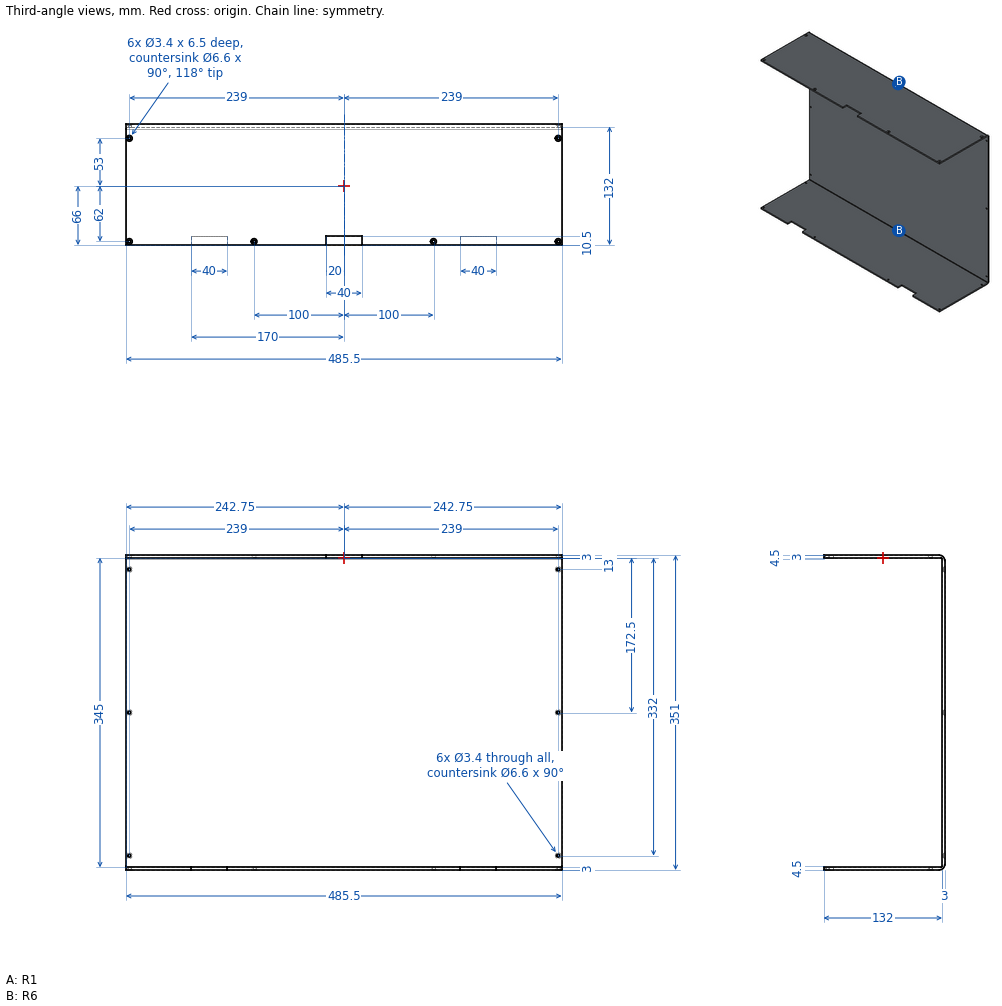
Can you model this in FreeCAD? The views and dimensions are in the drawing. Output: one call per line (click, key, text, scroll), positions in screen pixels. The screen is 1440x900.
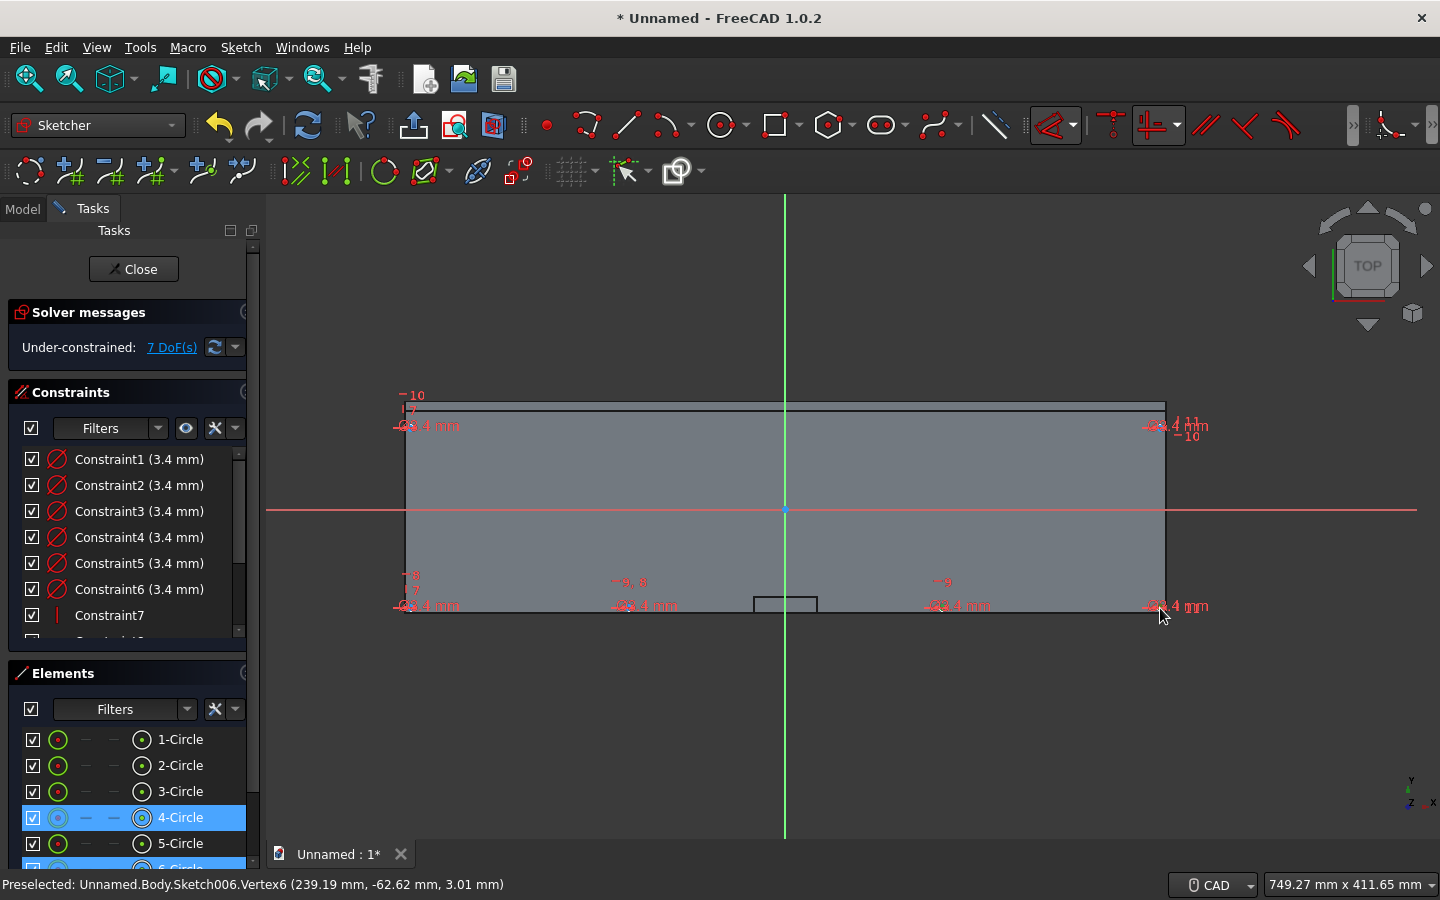
key(h)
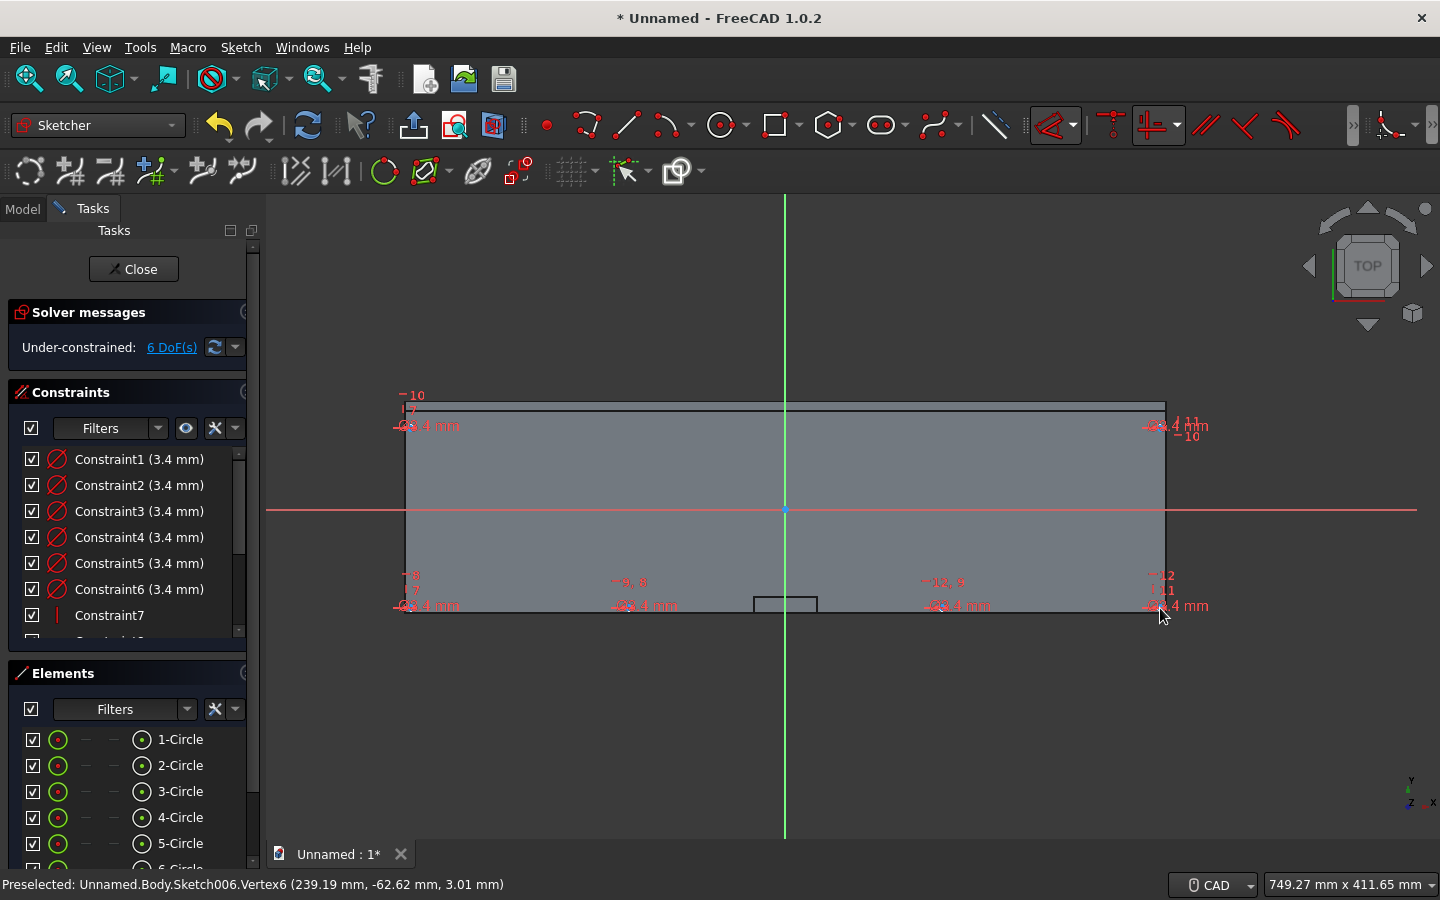
click(411, 428)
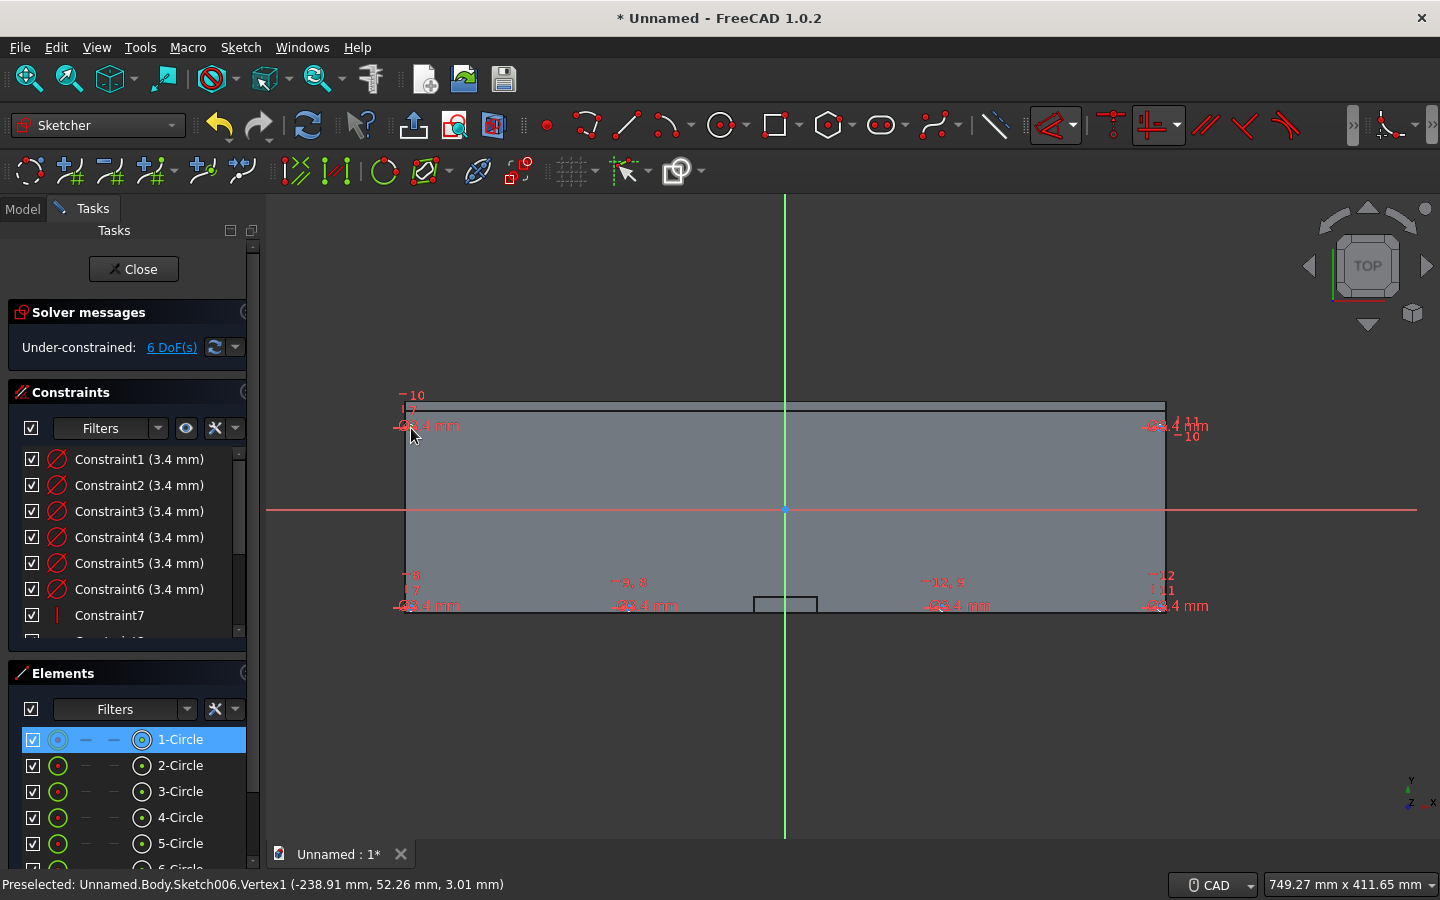
click(1076, 126)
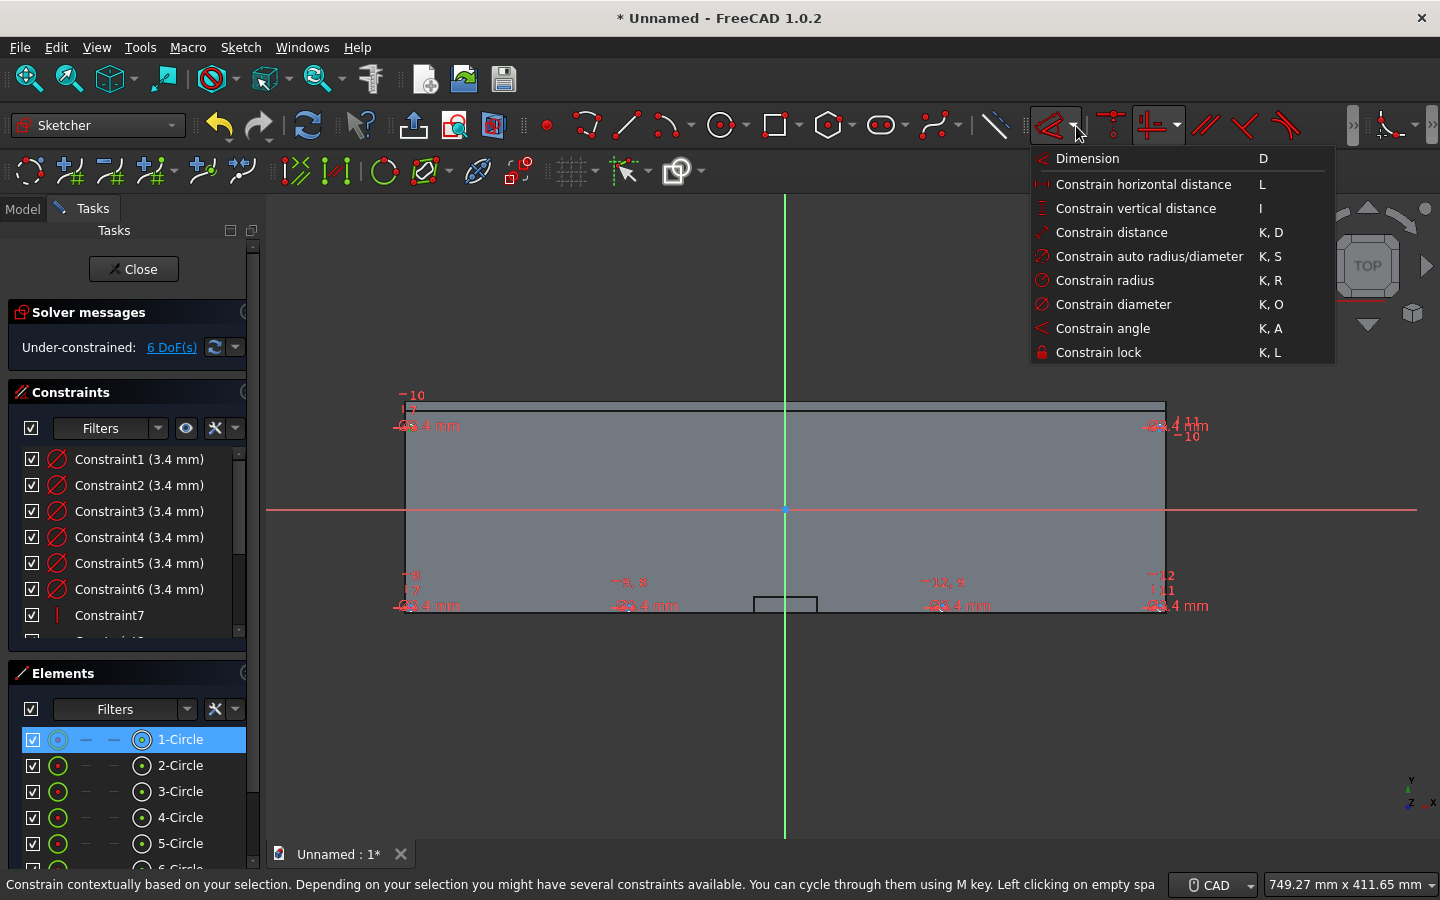
click(1183, 208)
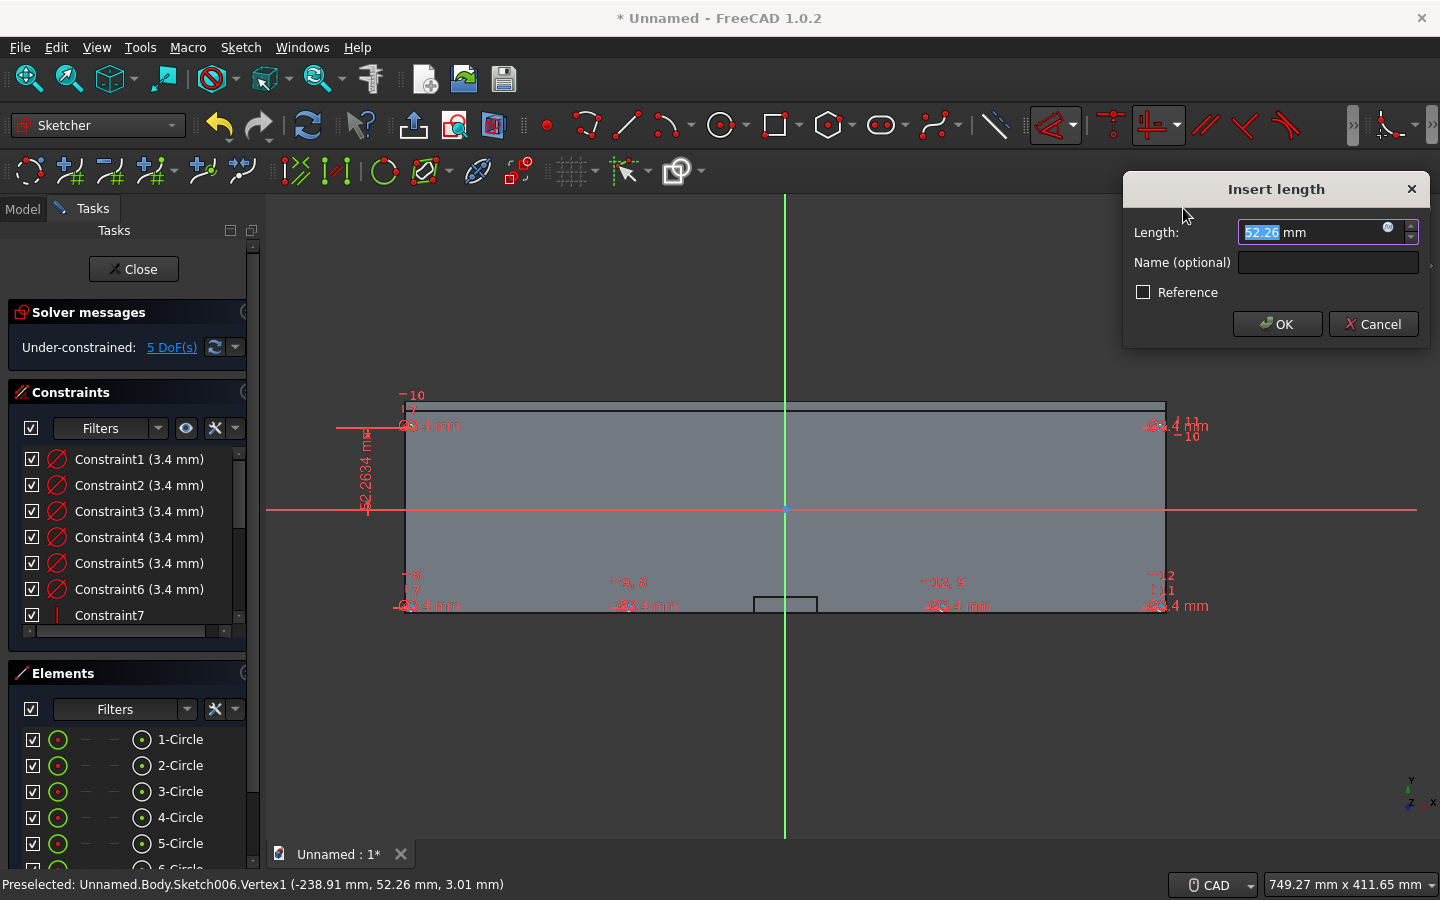
text(53)
key(Return)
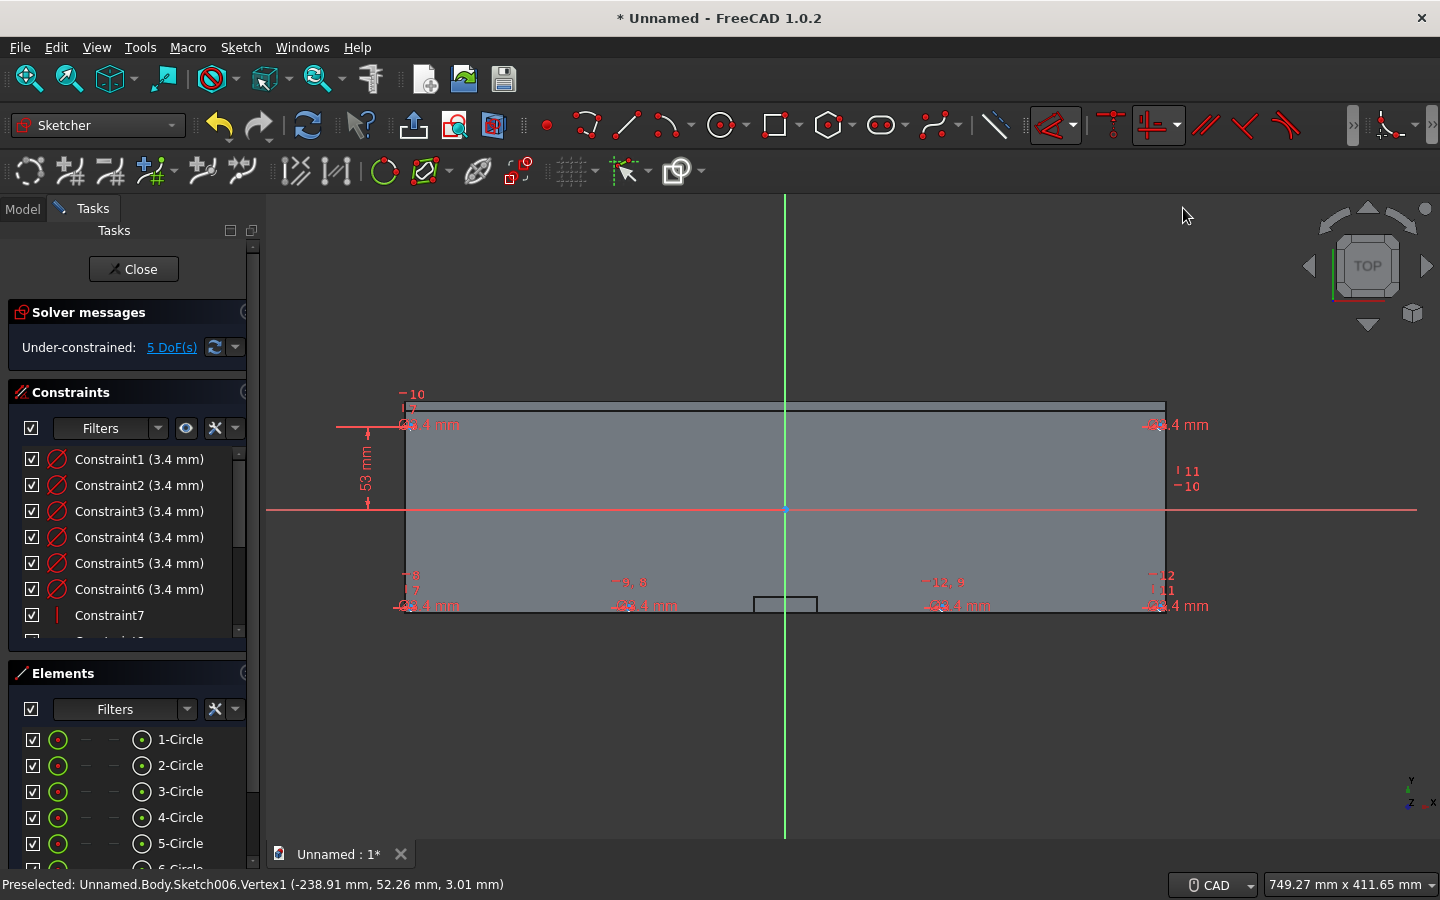
click(411, 608)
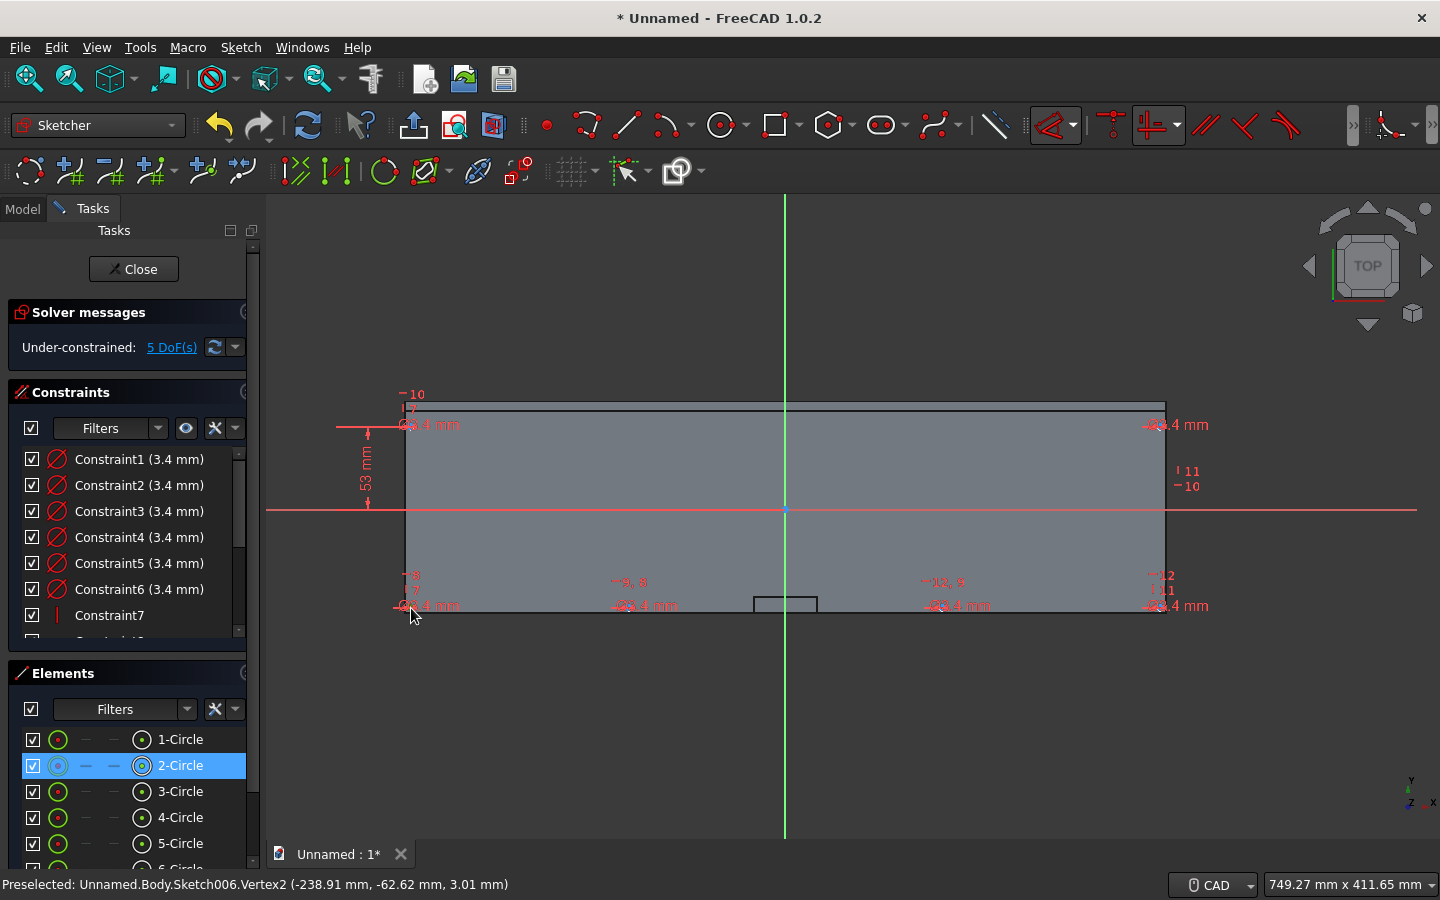
click(1076, 126)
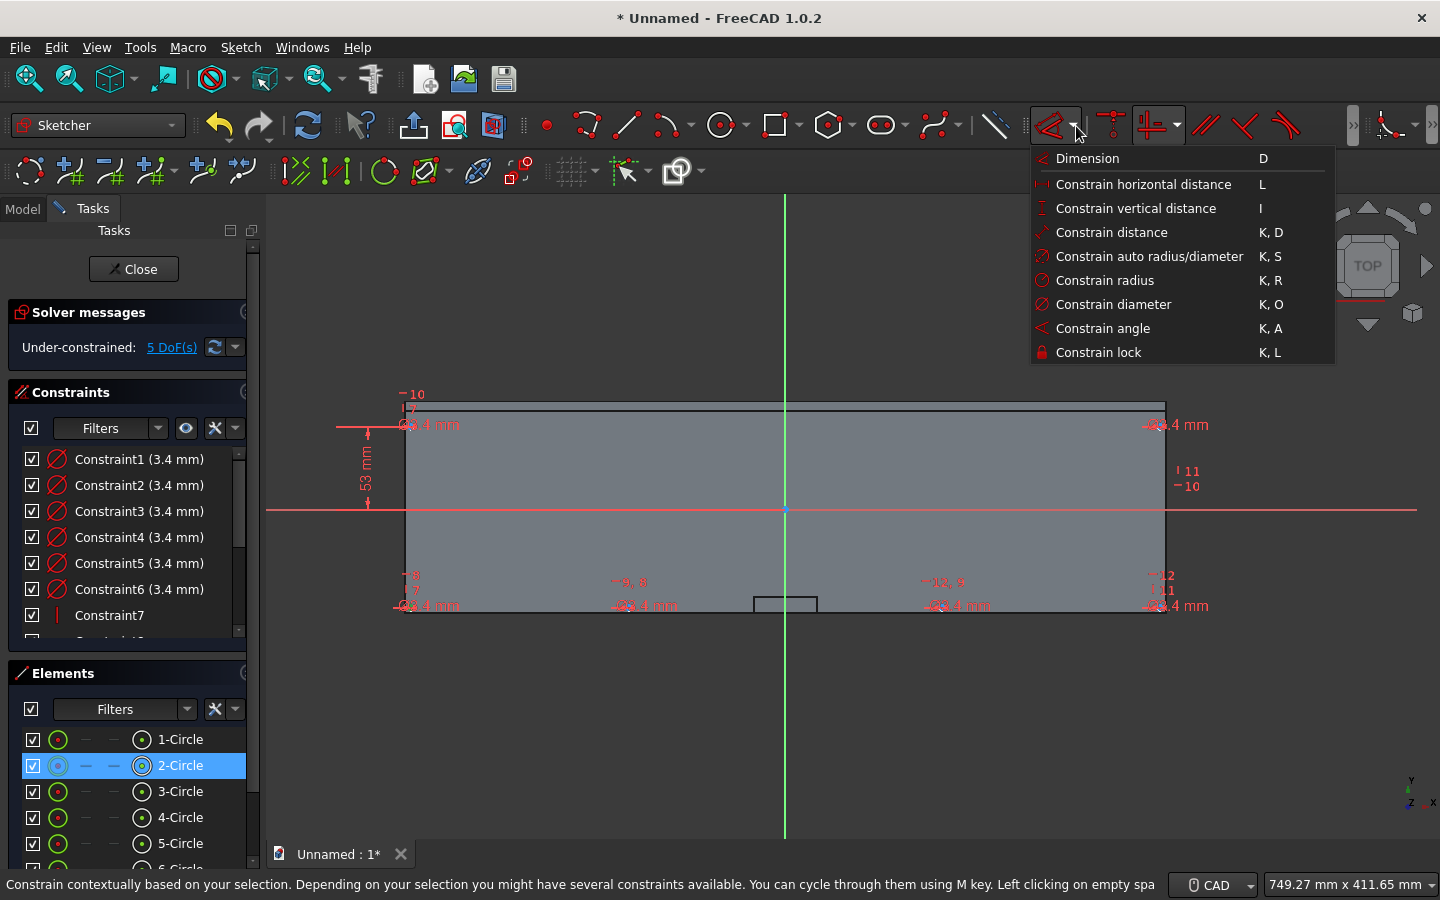
click(1183, 208)